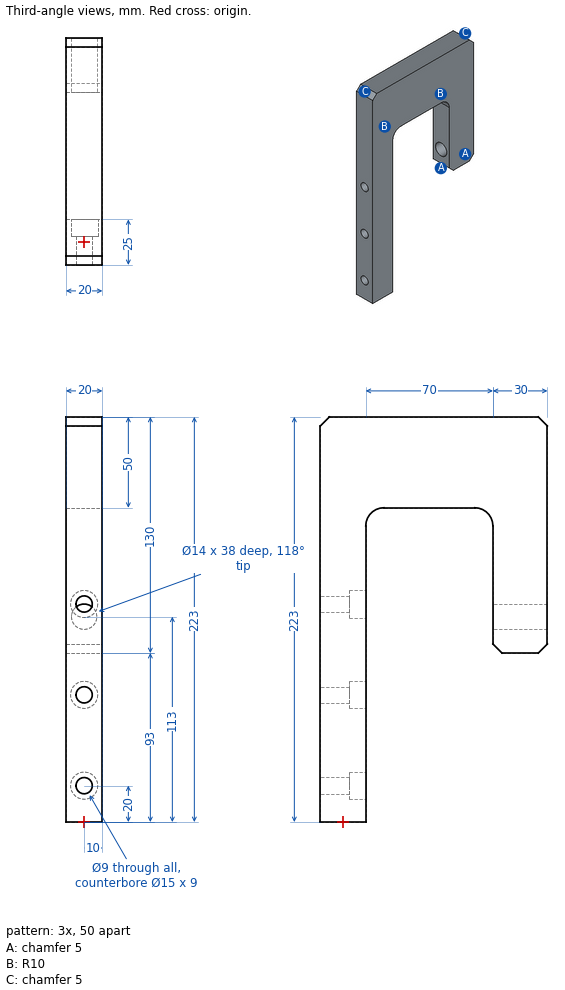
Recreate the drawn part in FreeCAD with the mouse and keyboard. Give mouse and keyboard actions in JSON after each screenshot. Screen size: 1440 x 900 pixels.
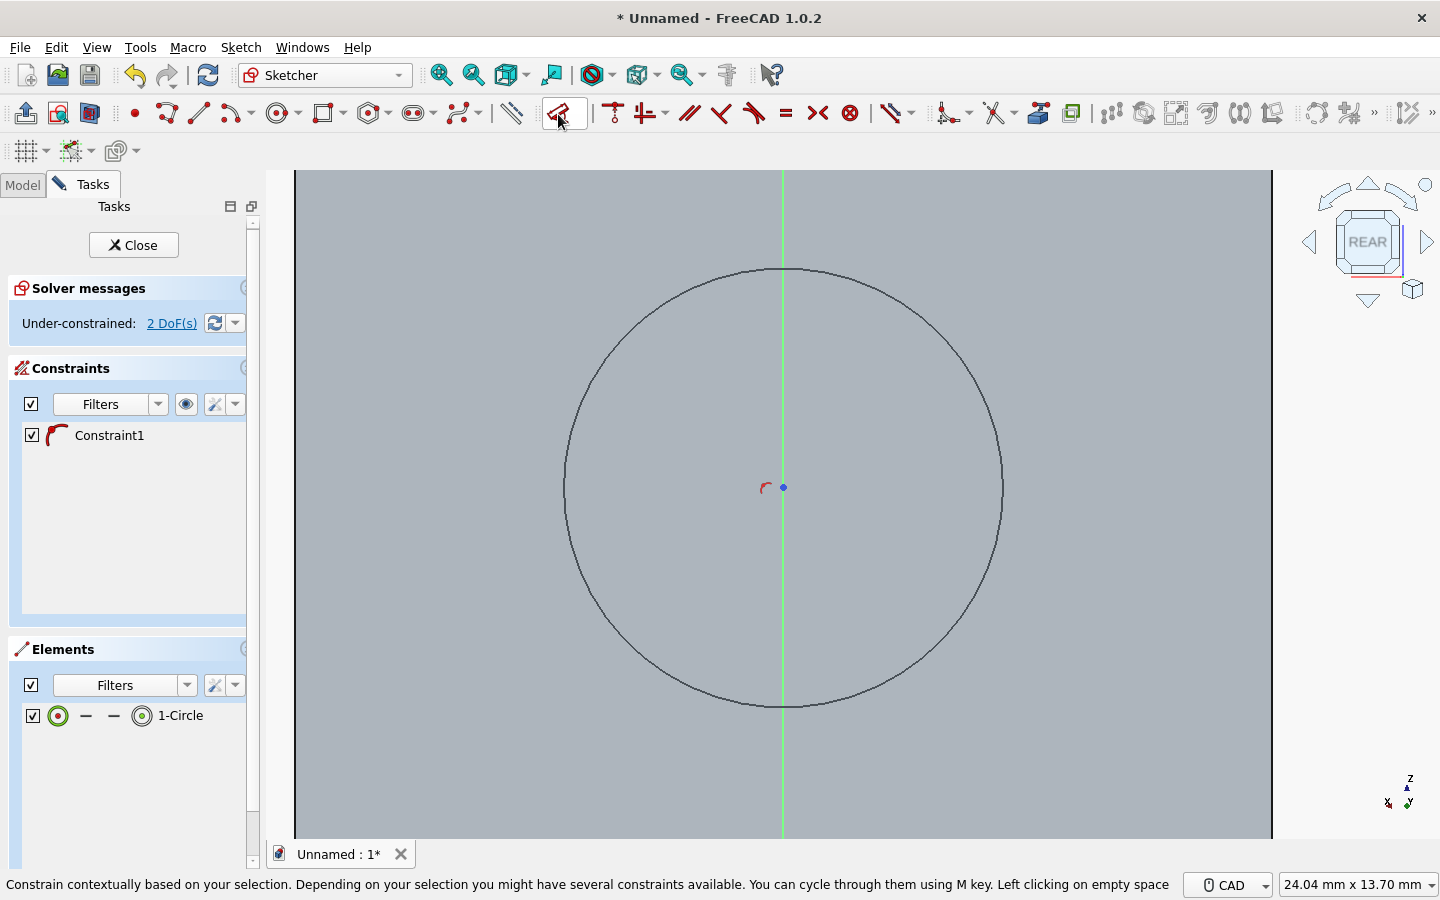
{"action": "left_click", "coordinate": [938, 332]}
{"action": "left_click", "coordinate": [961, 309]}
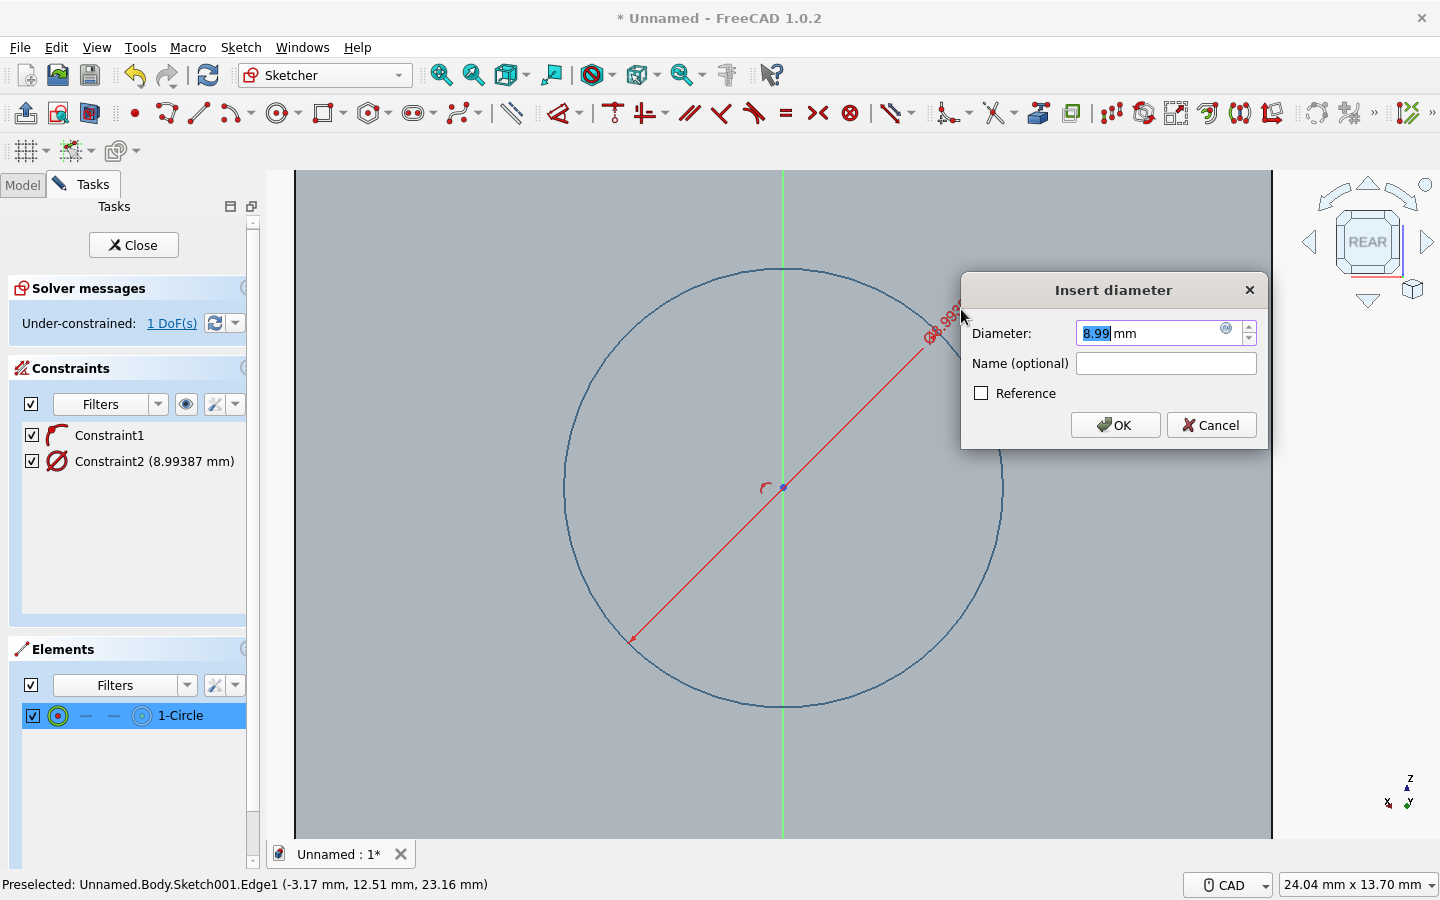
{"action": "type", "text": "9"}
{"action": "key", "text": "Return"}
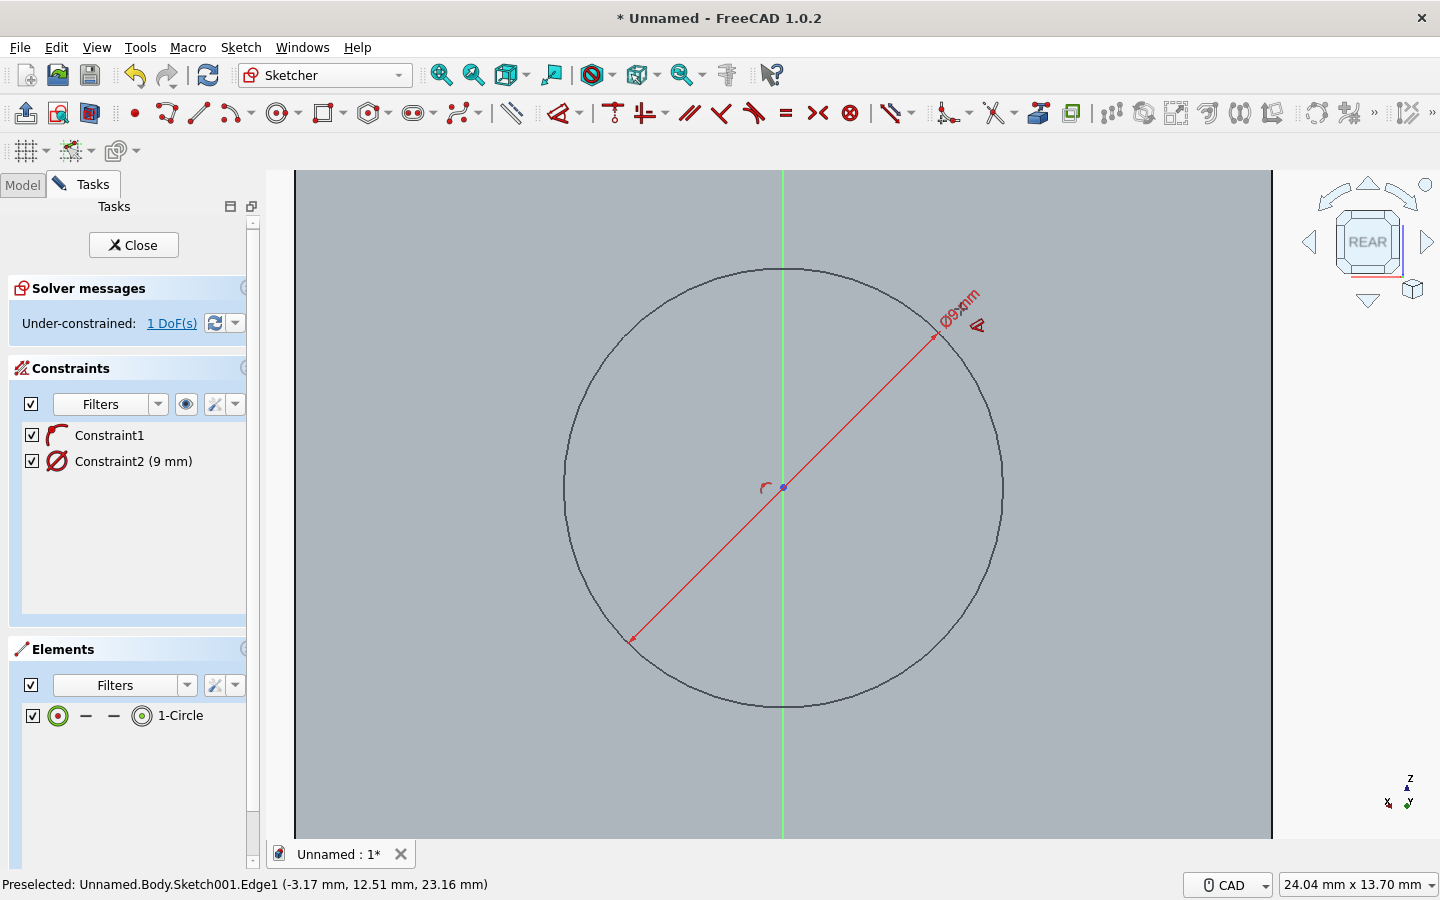
{"action": "left_click", "coordinate": [783, 488]}
{"action": "left_click", "coordinate": [817, 650]}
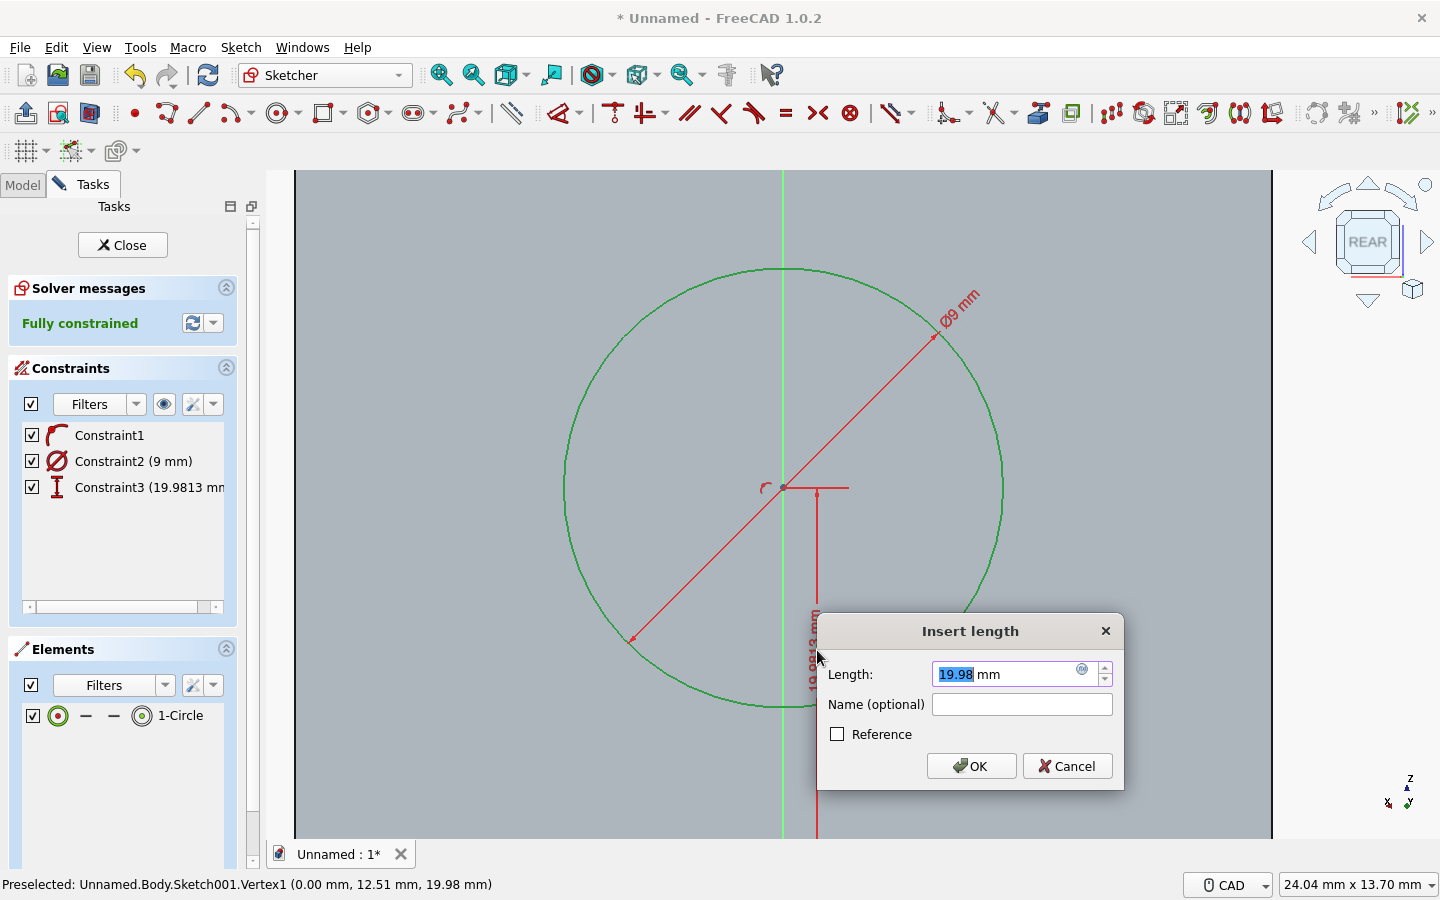
{"action": "type", "text": "20"}
{"action": "key", "text": "Return"}
{"action": "key", "text": "Escape"}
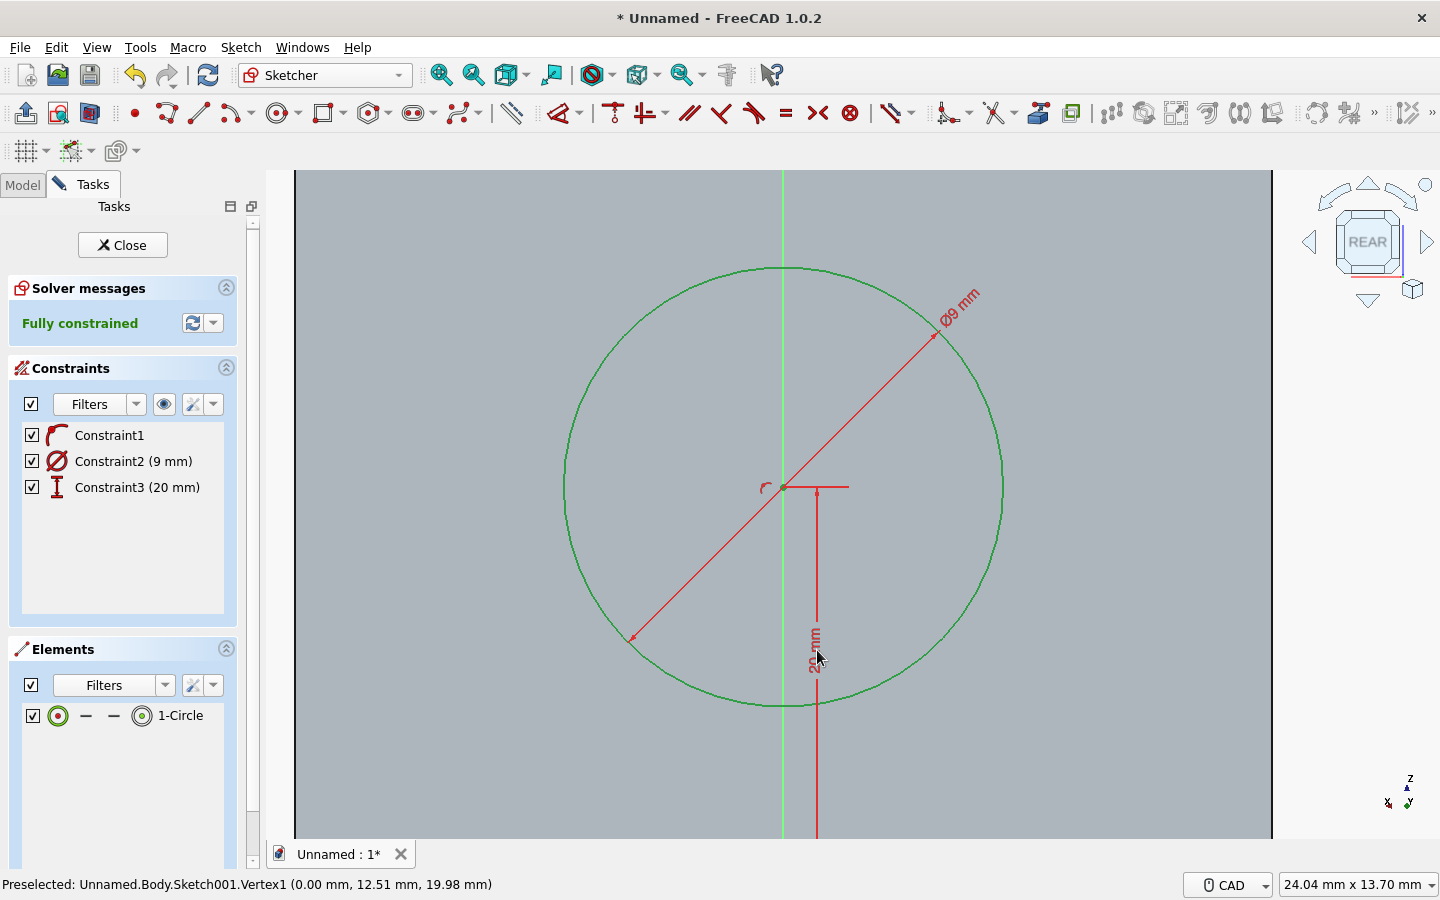
{"action": "left_click", "coordinate": [123, 245]}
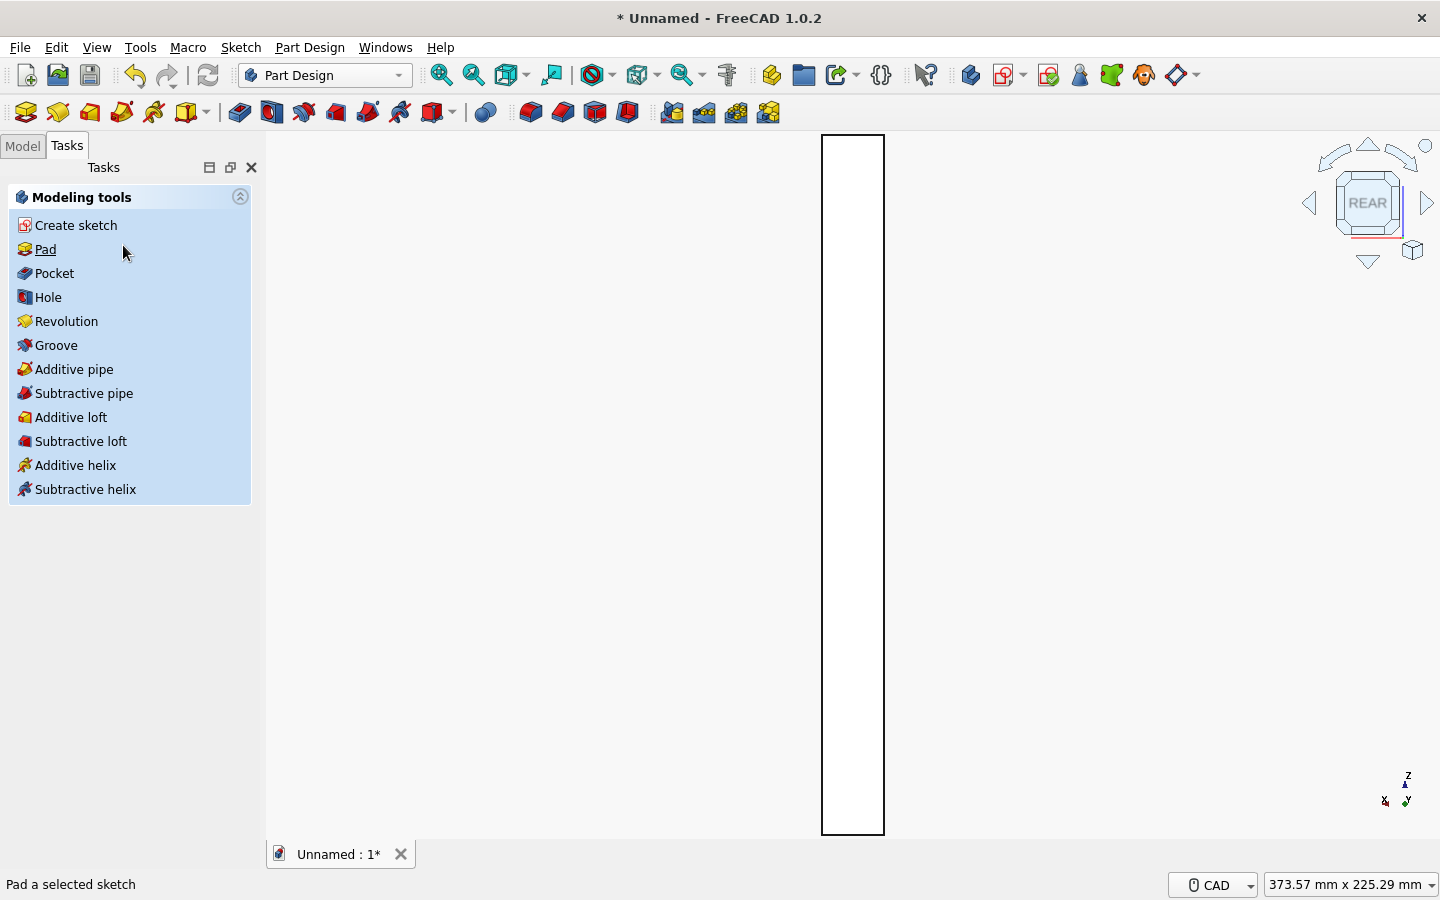
{"action": "left_click", "coordinate": [272, 112]}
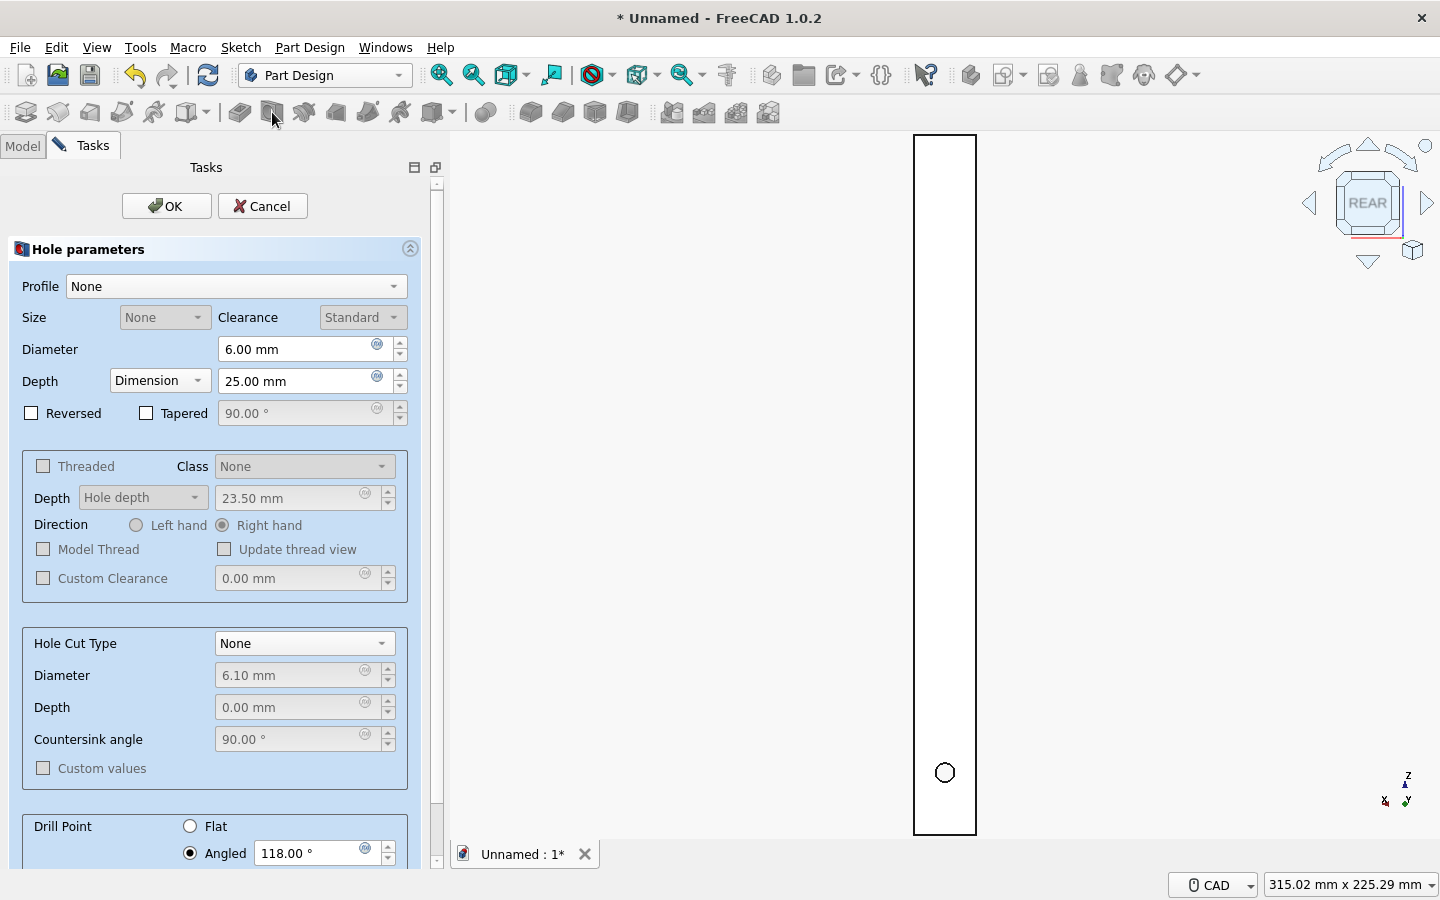
{"action": "triple_click", "coordinate": [305, 349]}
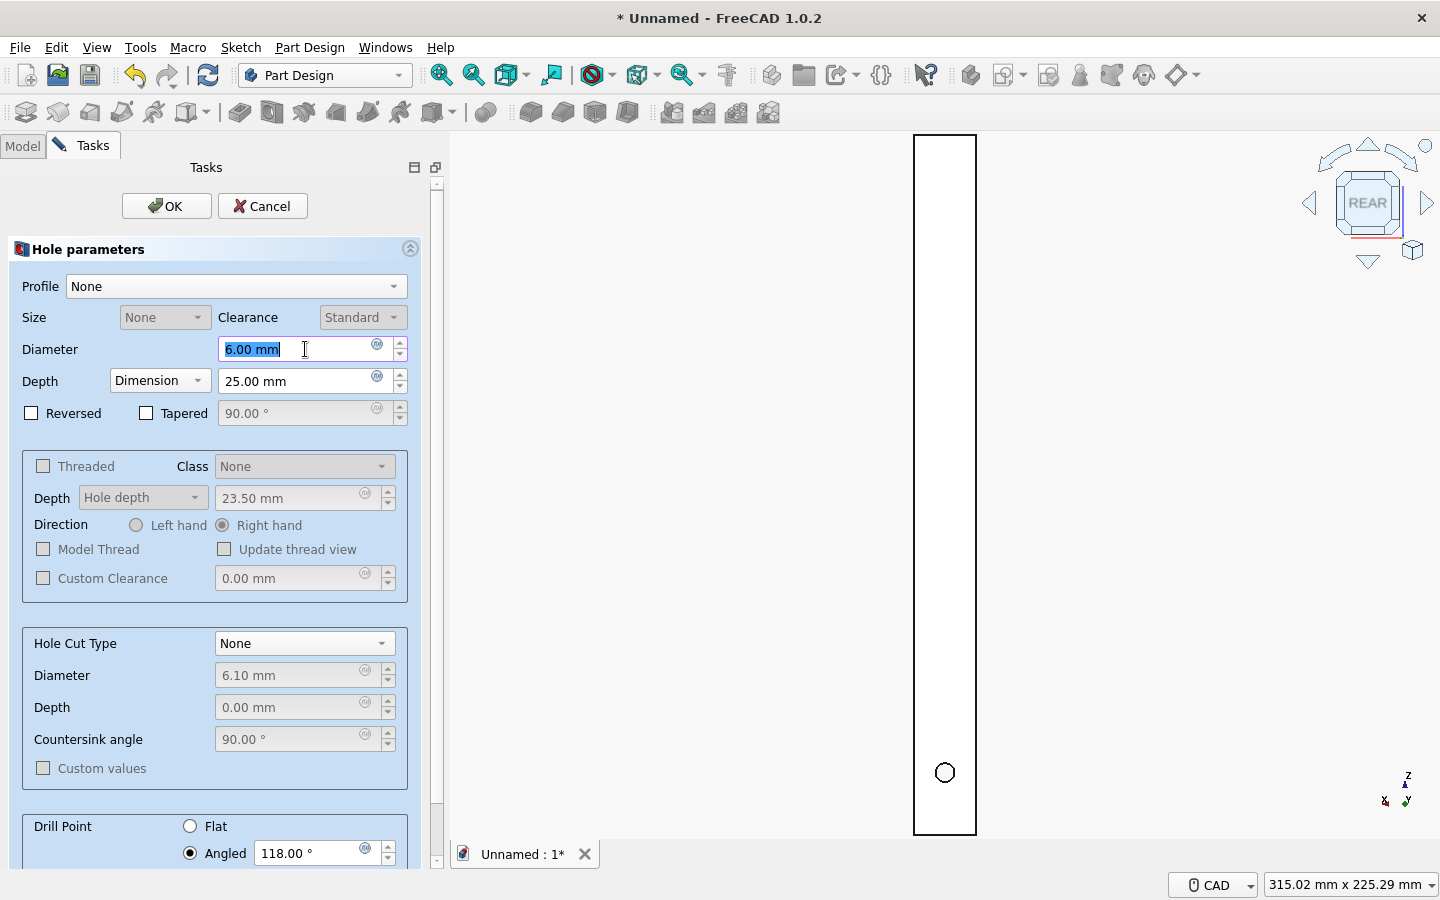
{"action": "type", "text": "9"}
{"action": "key", "text": "Tab"}